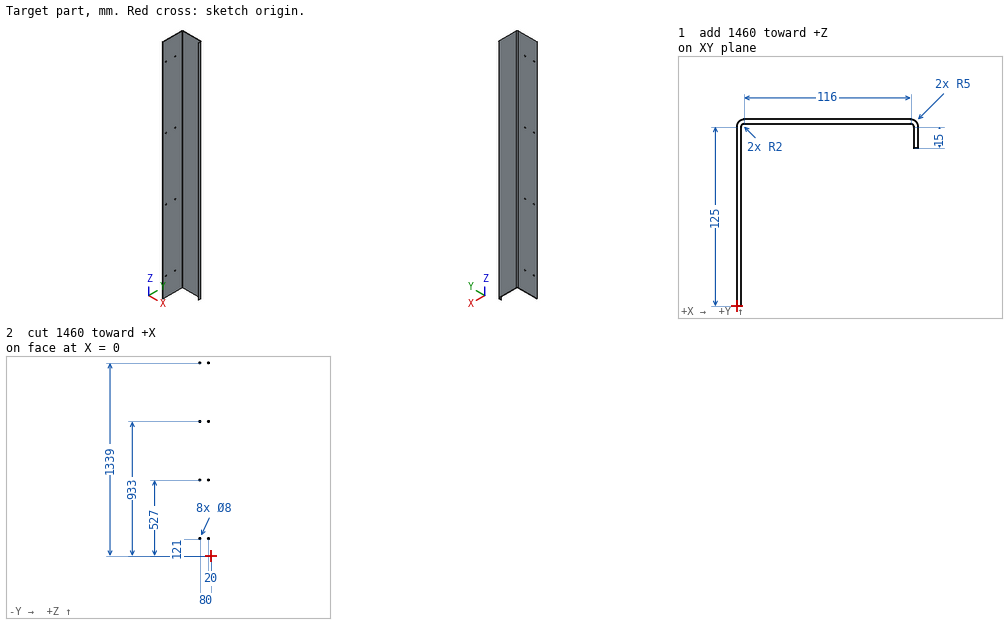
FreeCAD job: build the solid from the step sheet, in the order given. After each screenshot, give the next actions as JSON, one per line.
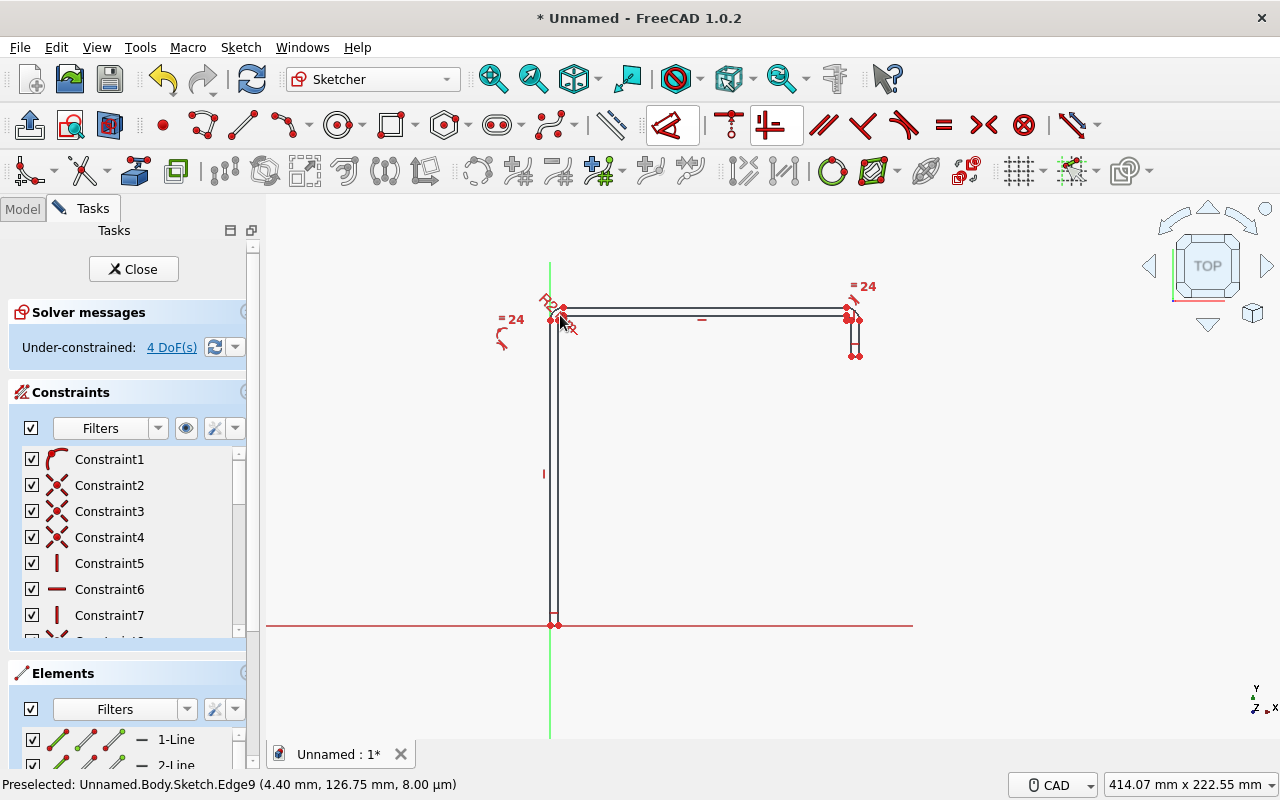
{"action": "scroll", "coordinate": [858, 315], "scroll_direction": "up", "scroll_amount": 6}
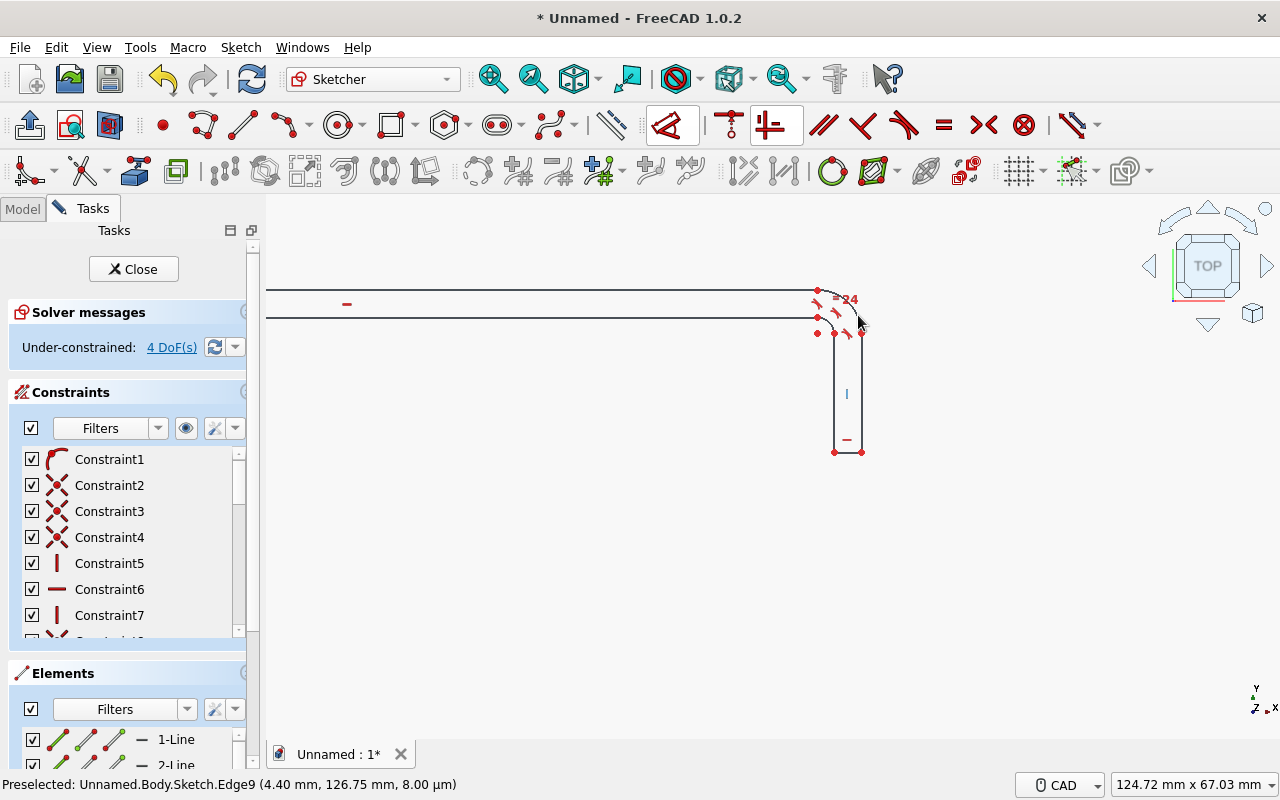
{"action": "left_click", "coordinate": [859, 320]}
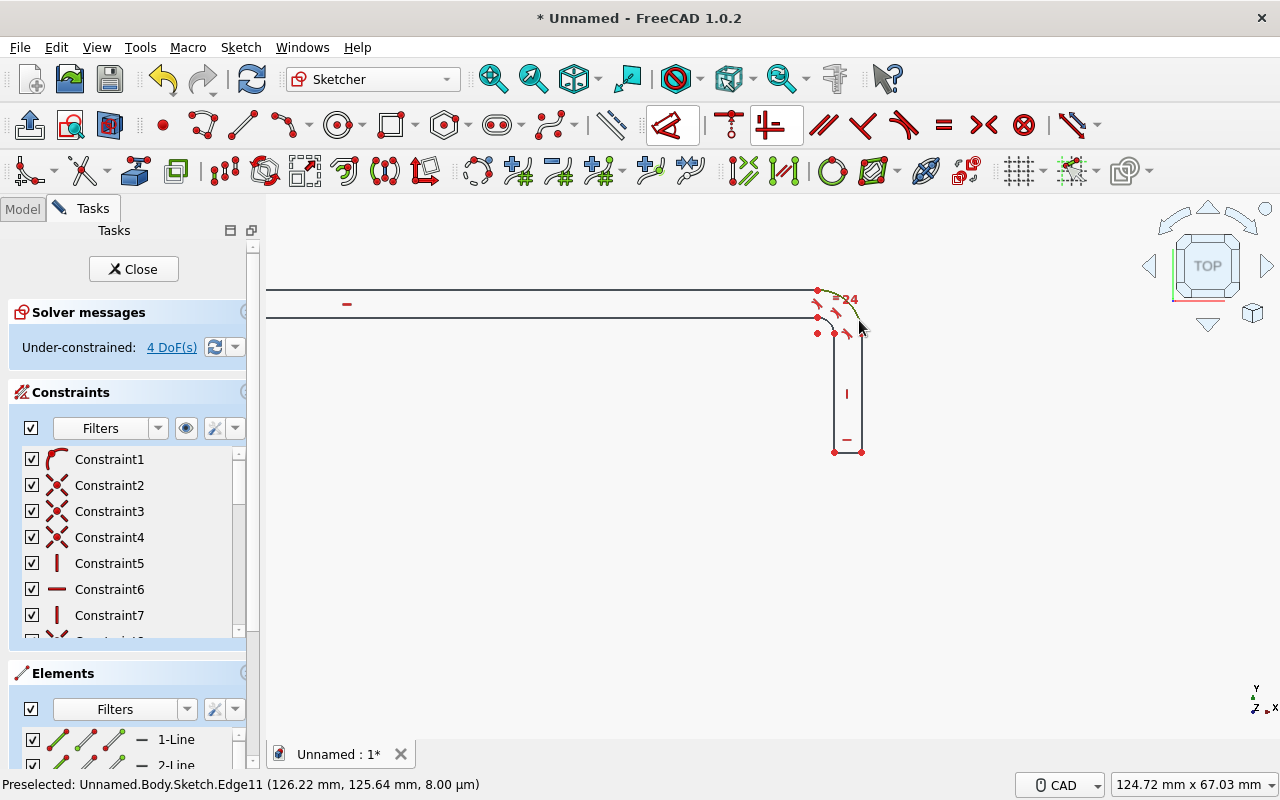
{"action": "key", "text": "k r"}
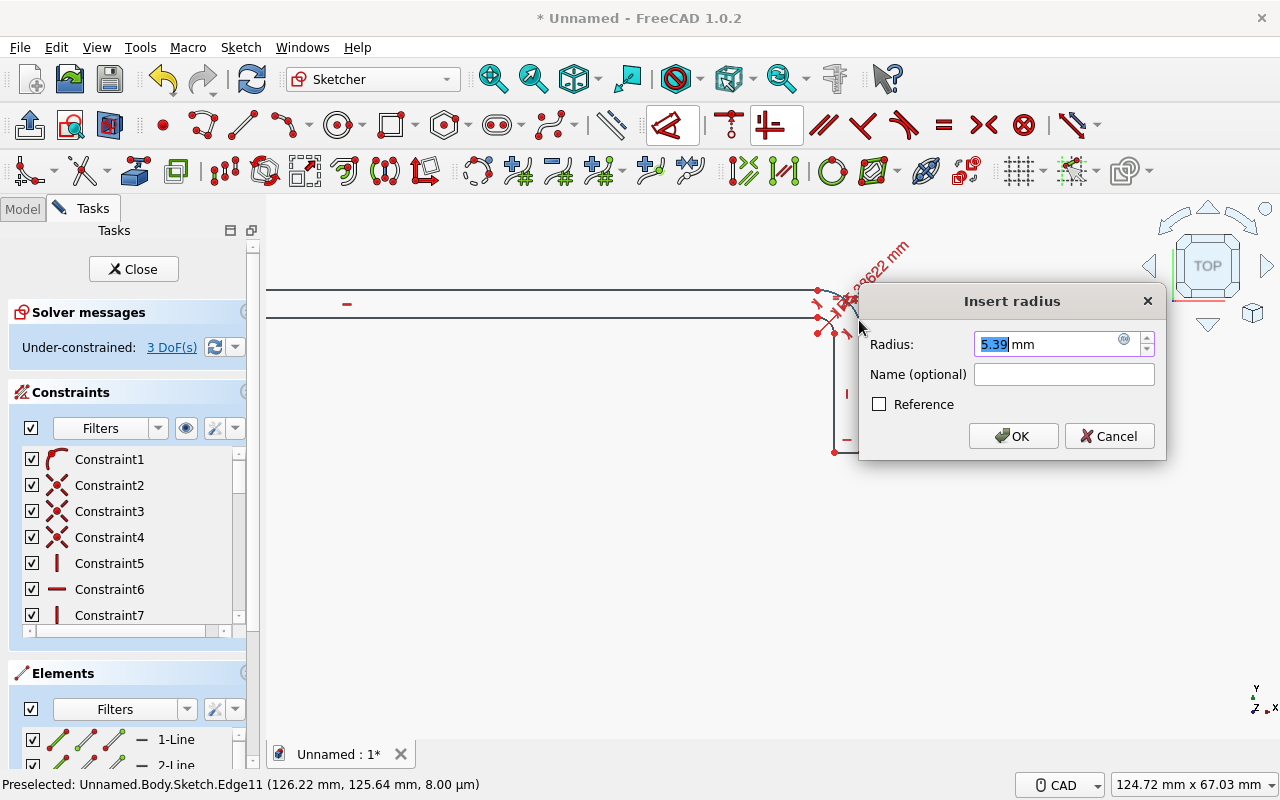
{"action": "type", "text": "5"}
{"action": "key", "text": "Return"}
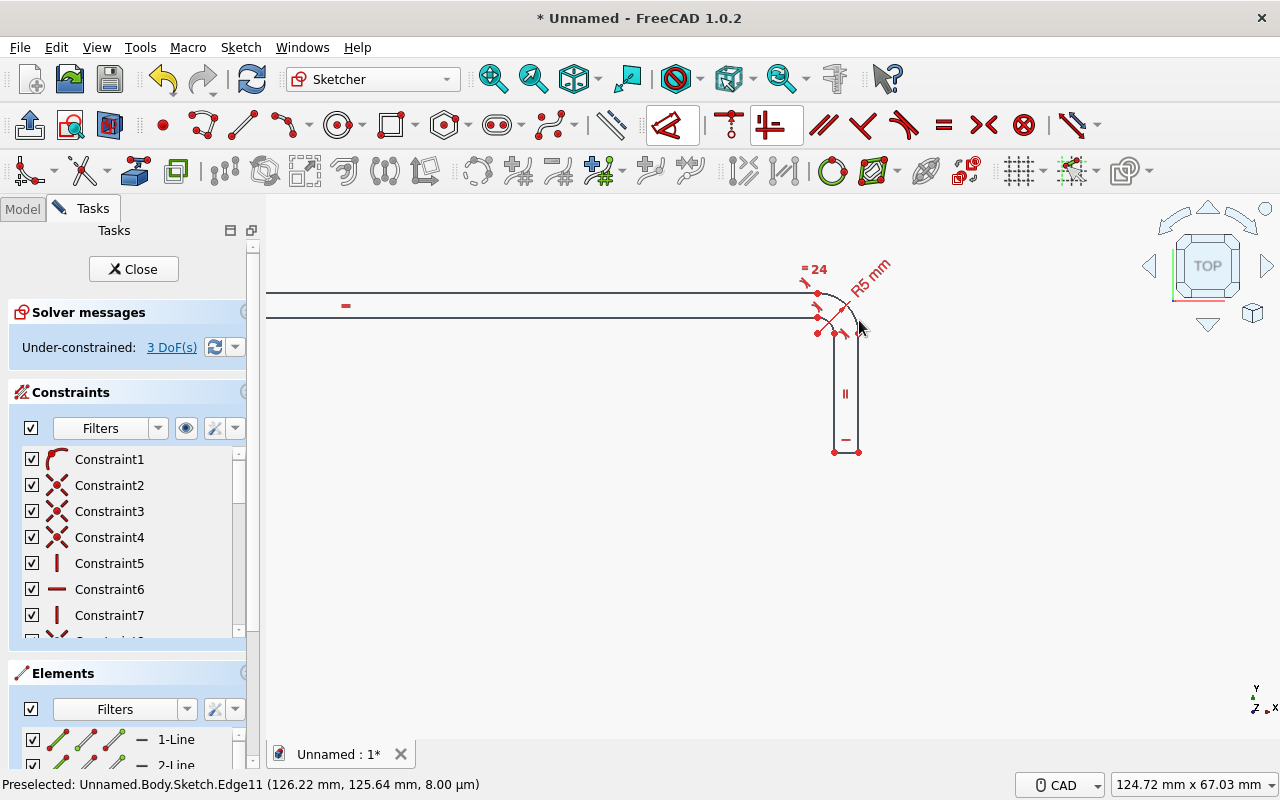
{"action": "left_click", "coordinate": [834, 370]}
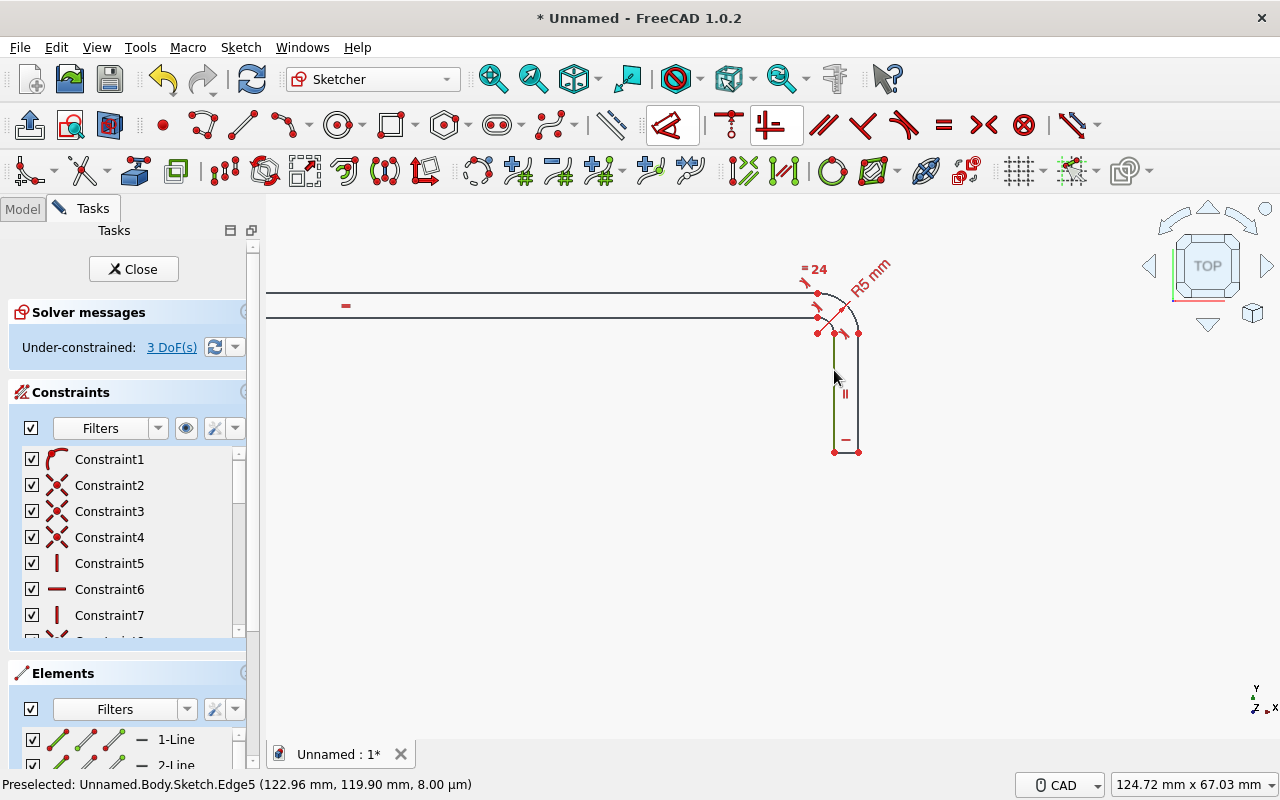
{"action": "key", "text": "i"}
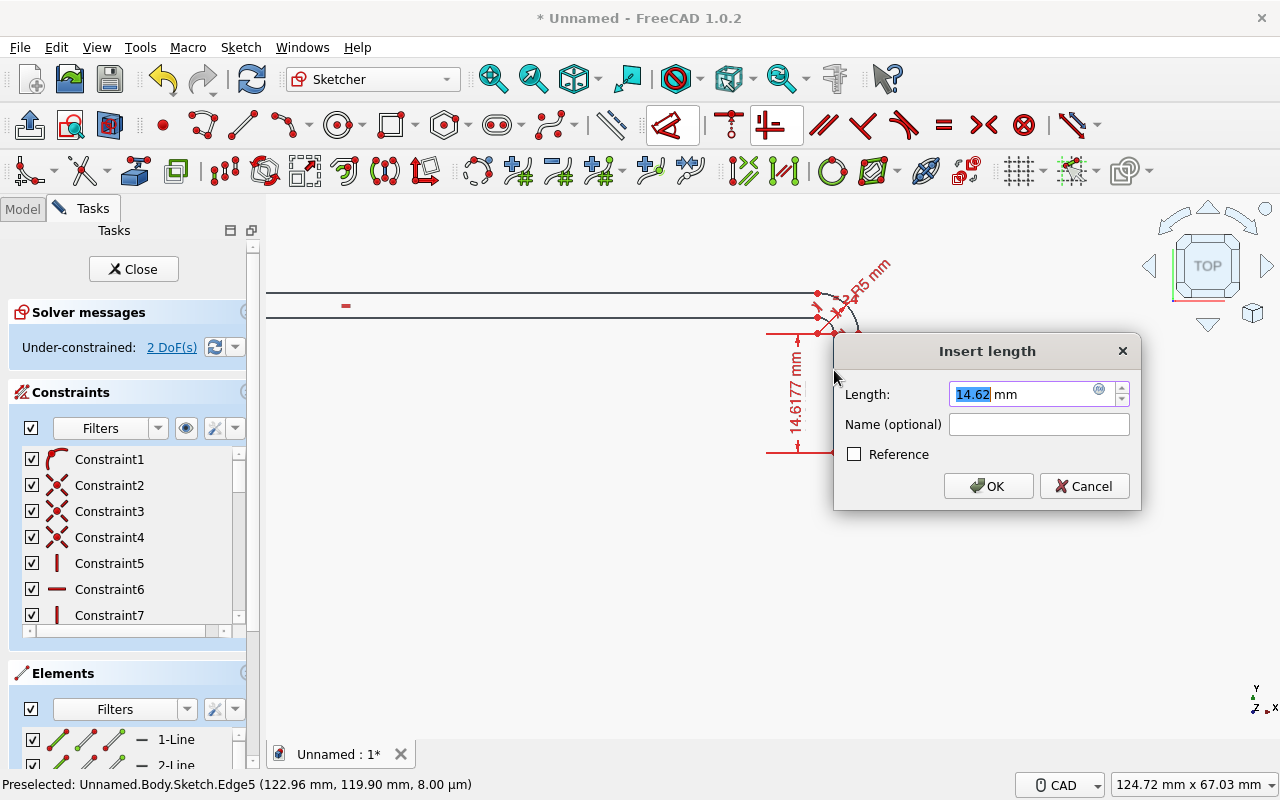
{"action": "type", "text": "15"}
{"action": "key", "text": "Return"}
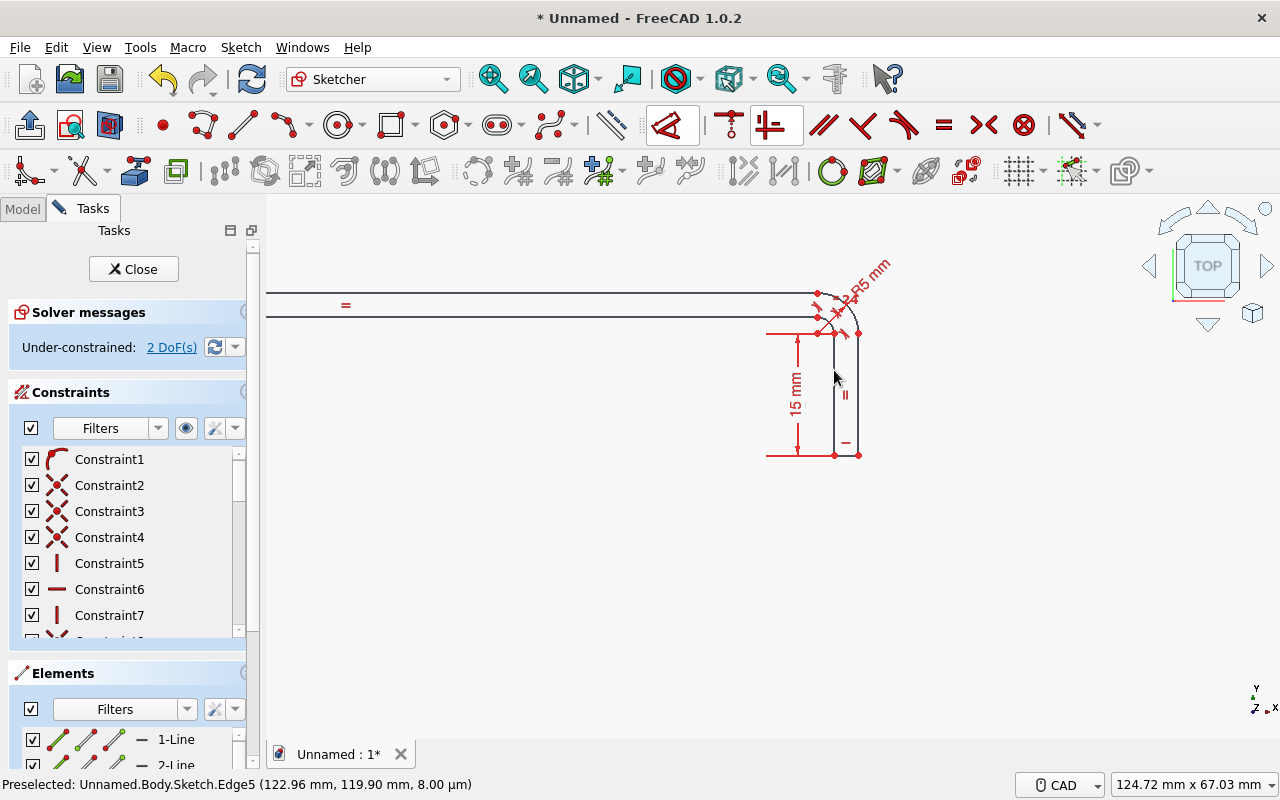
{"action": "scroll", "coordinate": [859, 315], "scroll_direction": "down", "scroll_amount": 6}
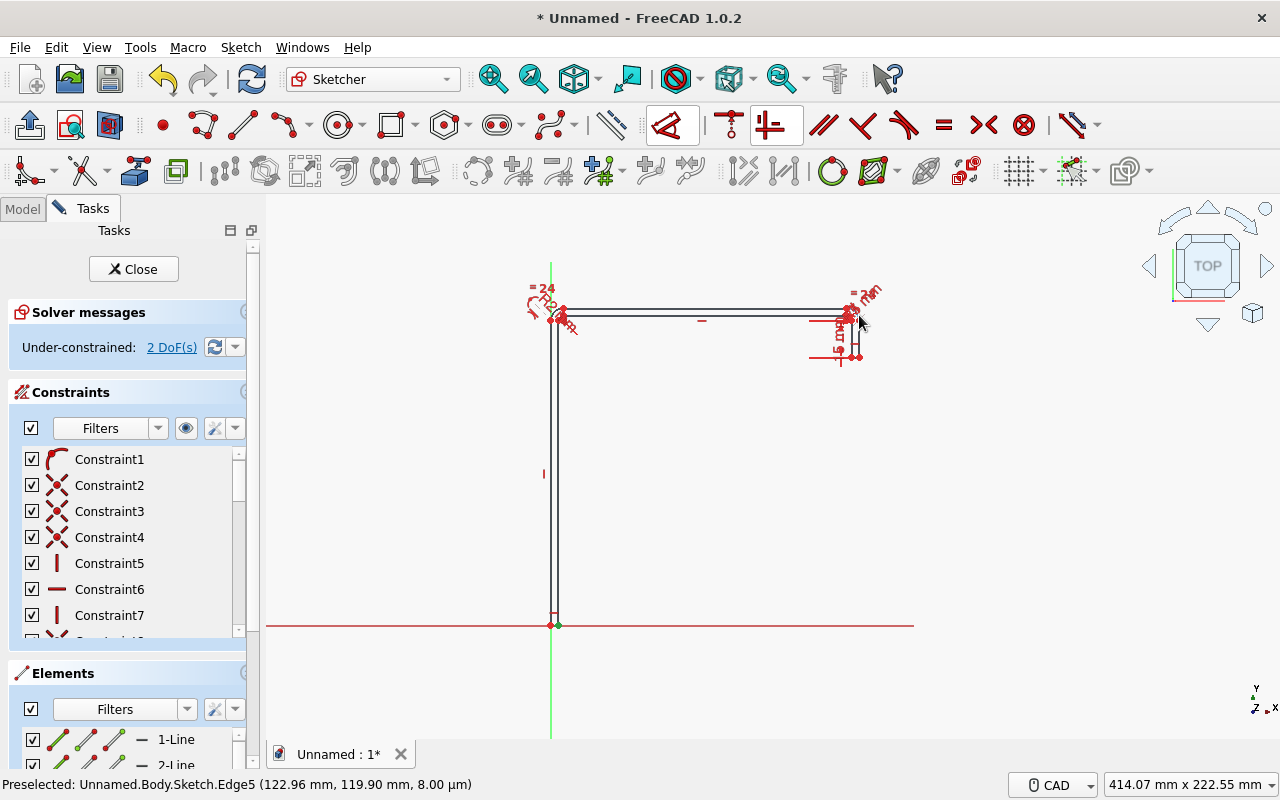
{"action": "scroll", "coordinate": [551, 412], "scroll_direction": "up", "scroll_amount": 4}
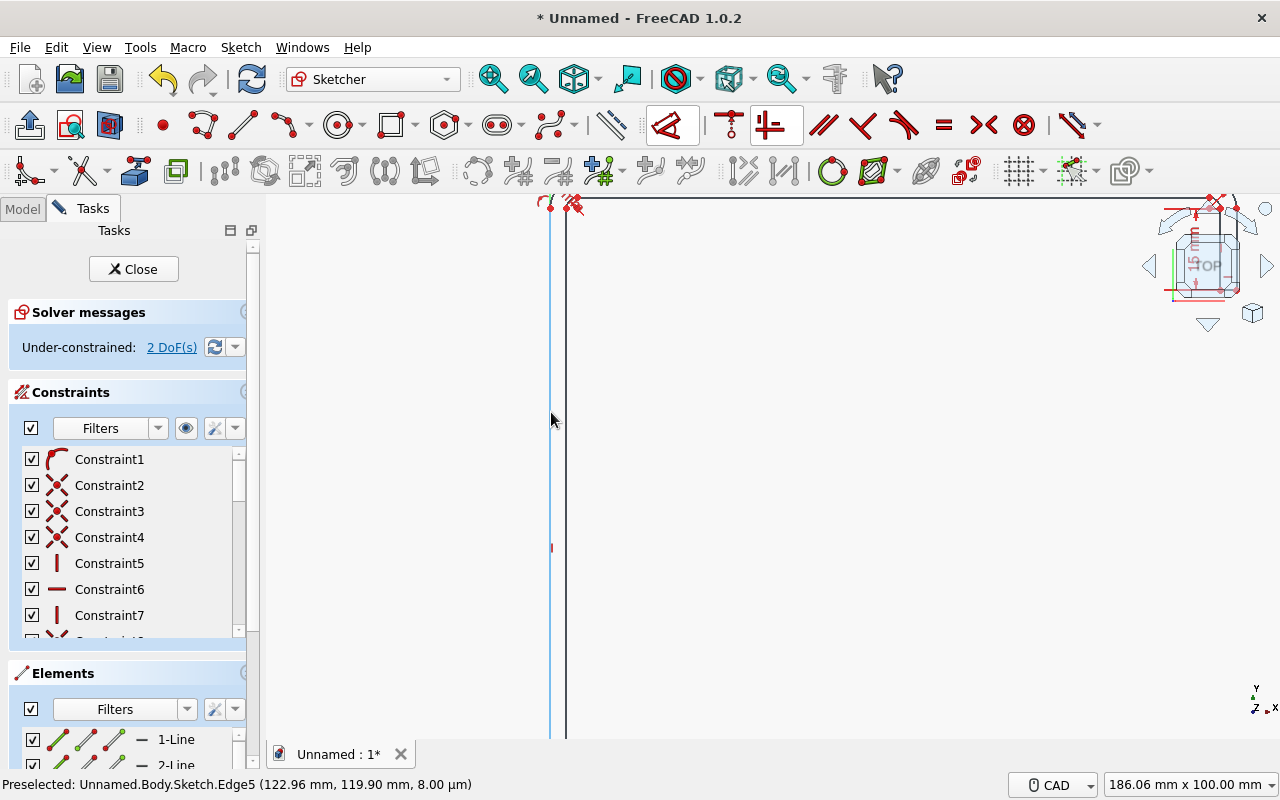
{"action": "left_click", "coordinate": [550, 412]}